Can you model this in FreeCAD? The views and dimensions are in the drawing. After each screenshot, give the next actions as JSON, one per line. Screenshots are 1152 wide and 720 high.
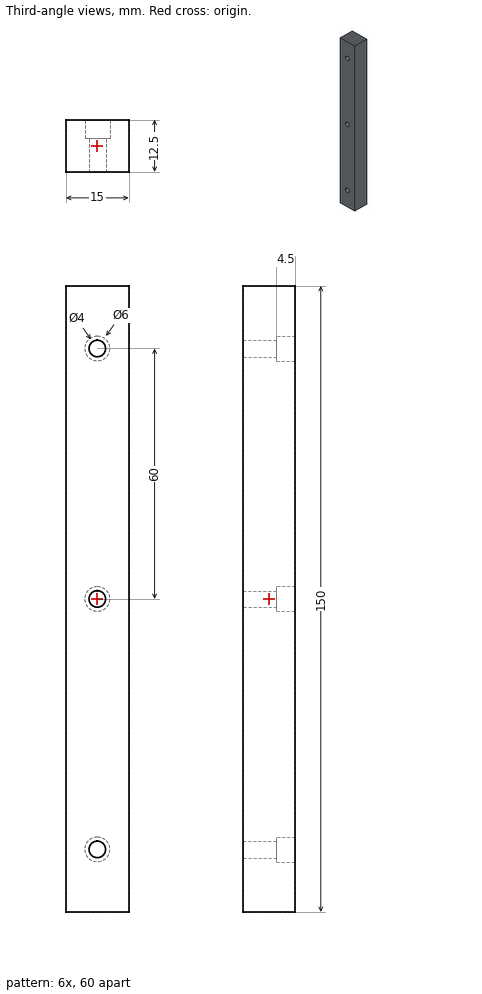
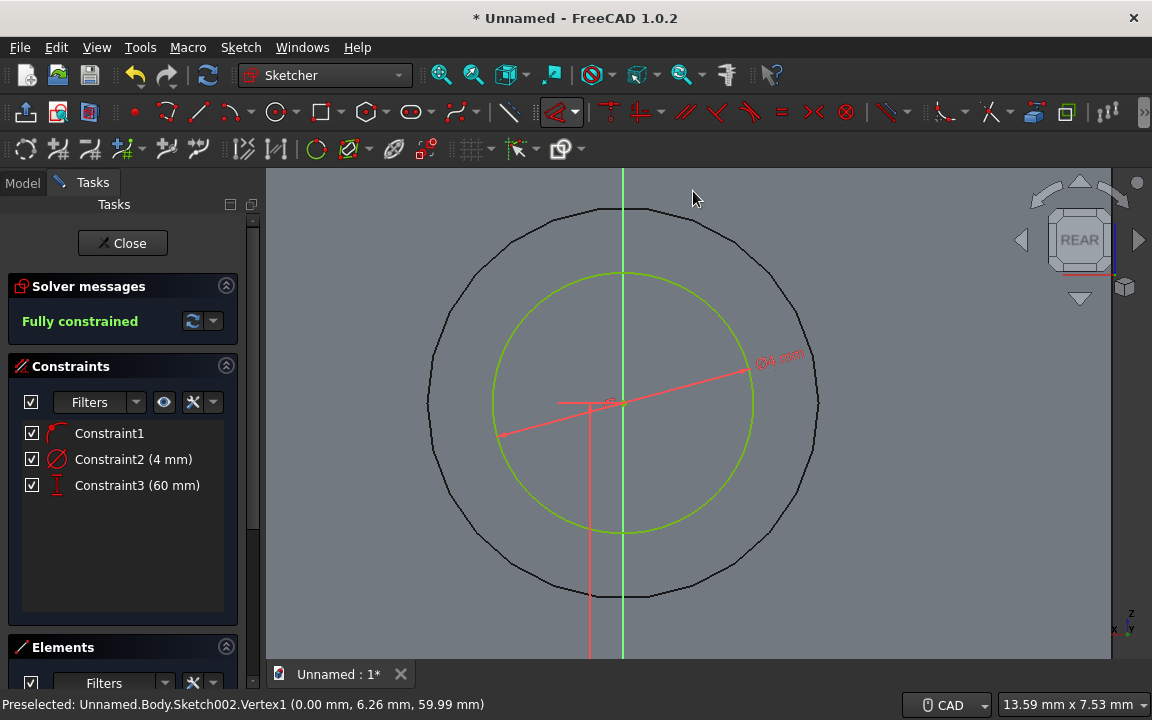
{"action": "left_click", "coordinate": [123, 243]}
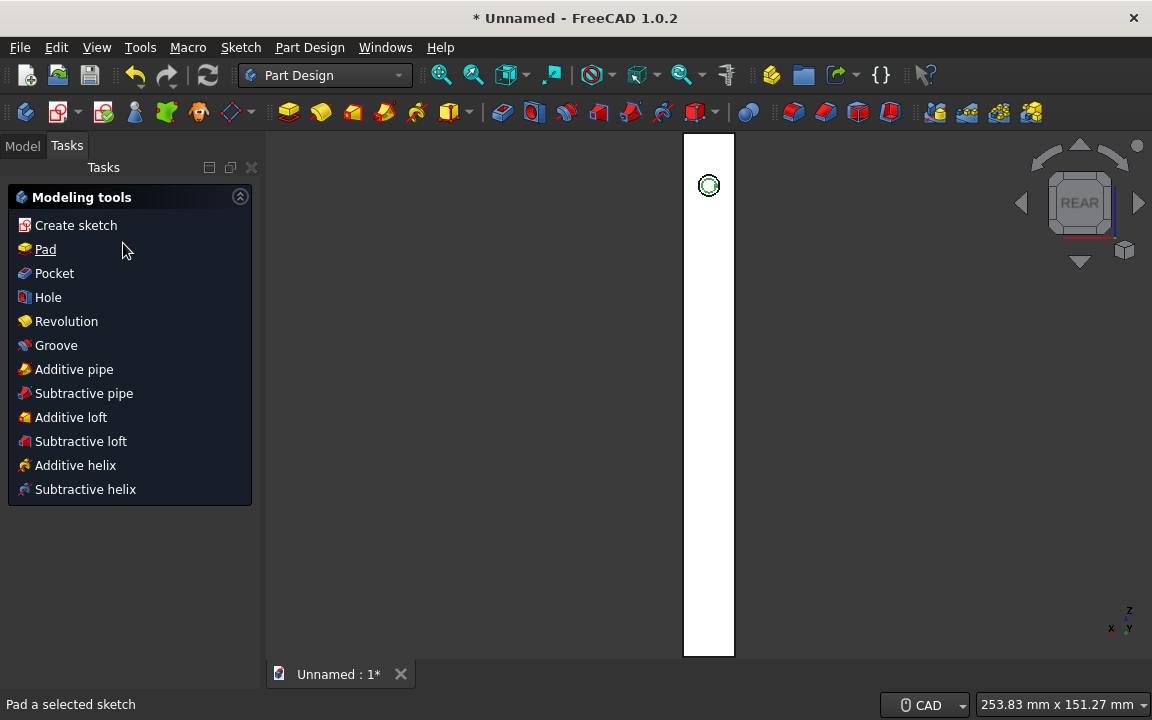
{"action": "left_click", "coordinate": [504, 112]}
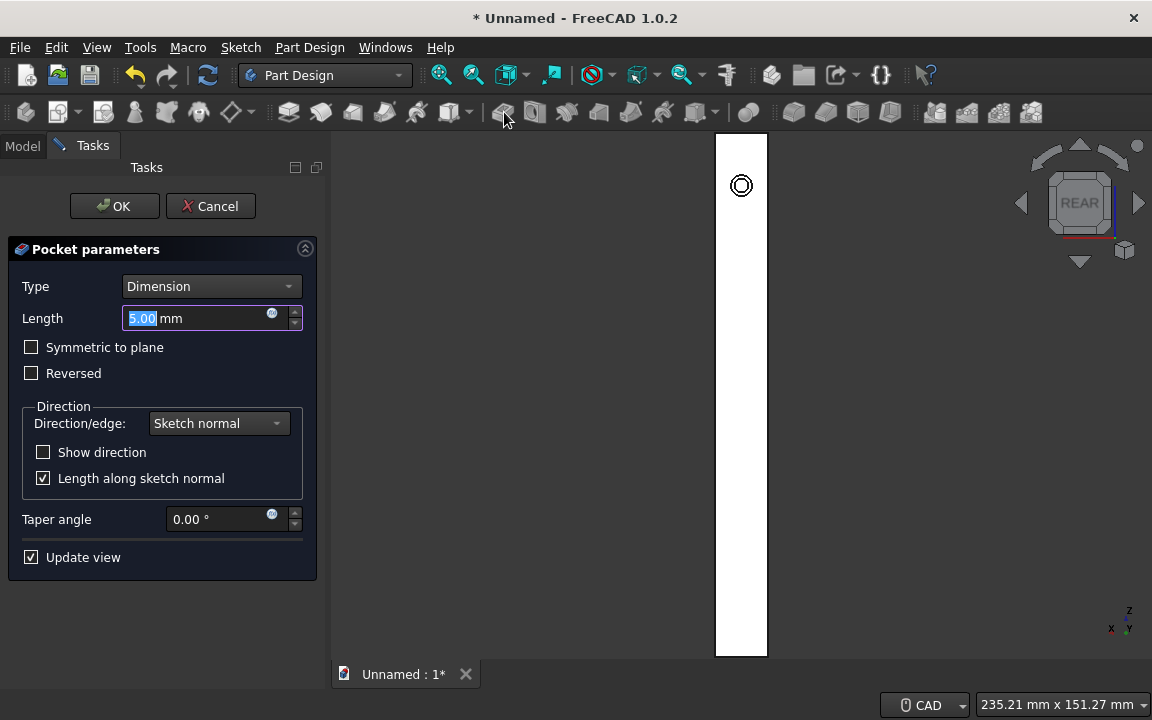
{"action": "left_click", "coordinate": [212, 286]}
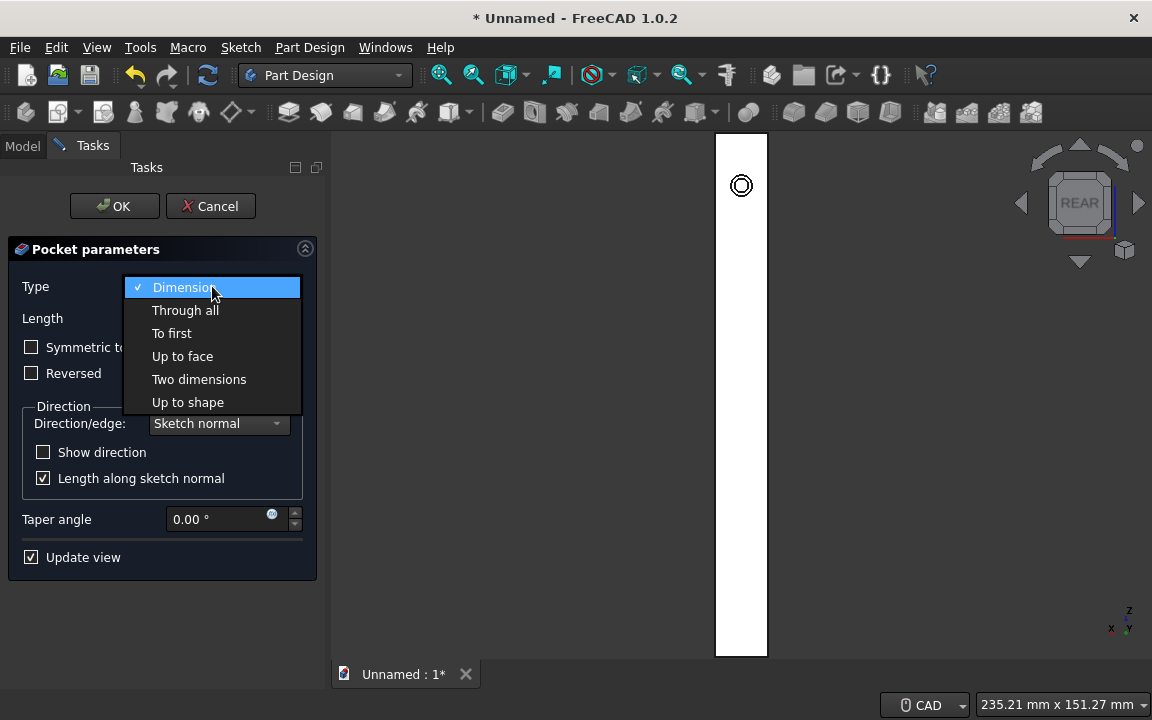
{"action": "left_click", "coordinate": [212, 310]}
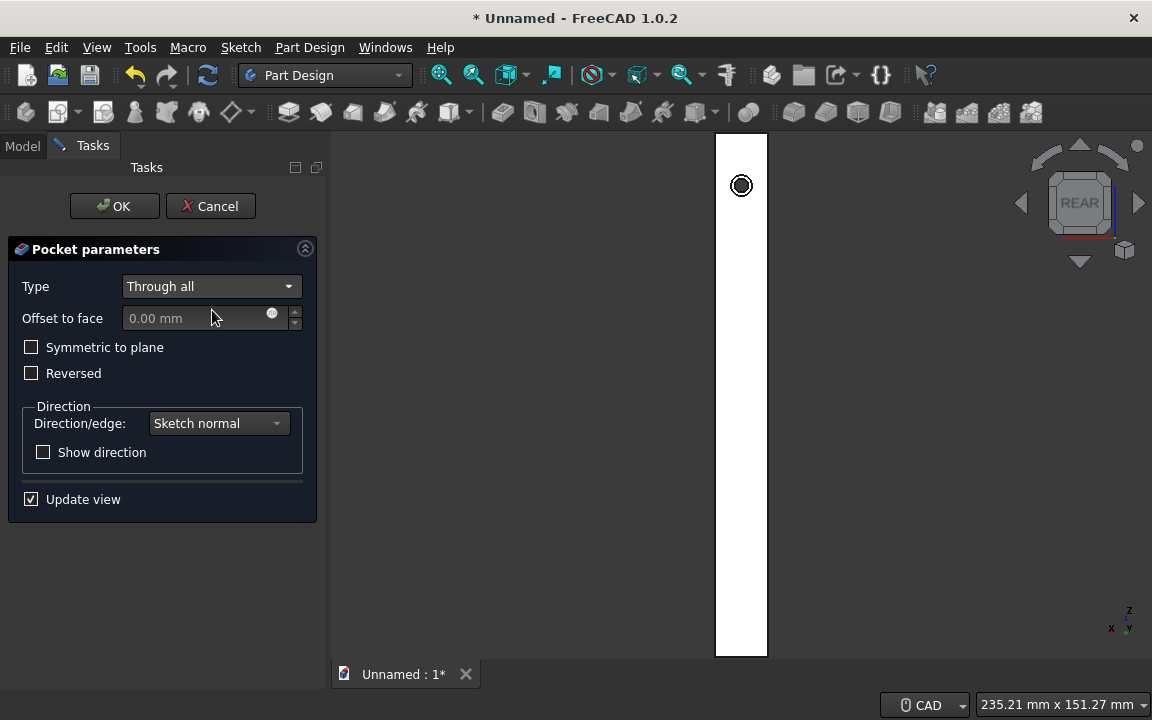
{"action": "left_click", "coordinate": [115, 206]}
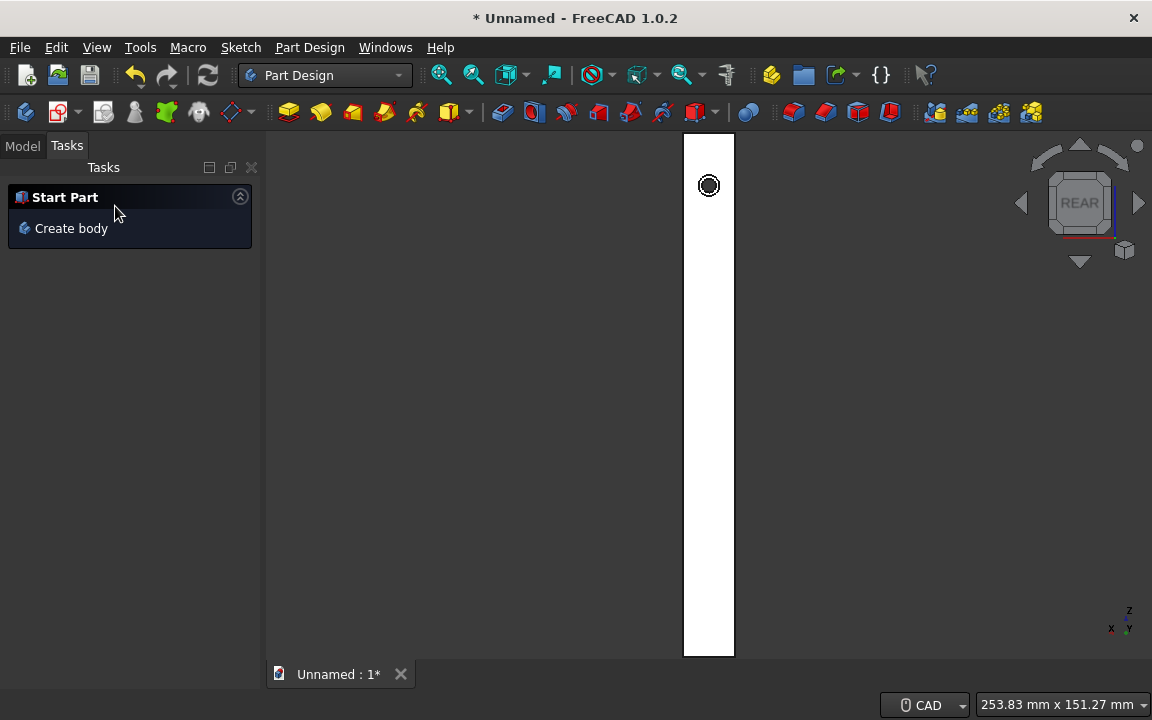
{"action": "left_click", "coordinate": [23, 145]}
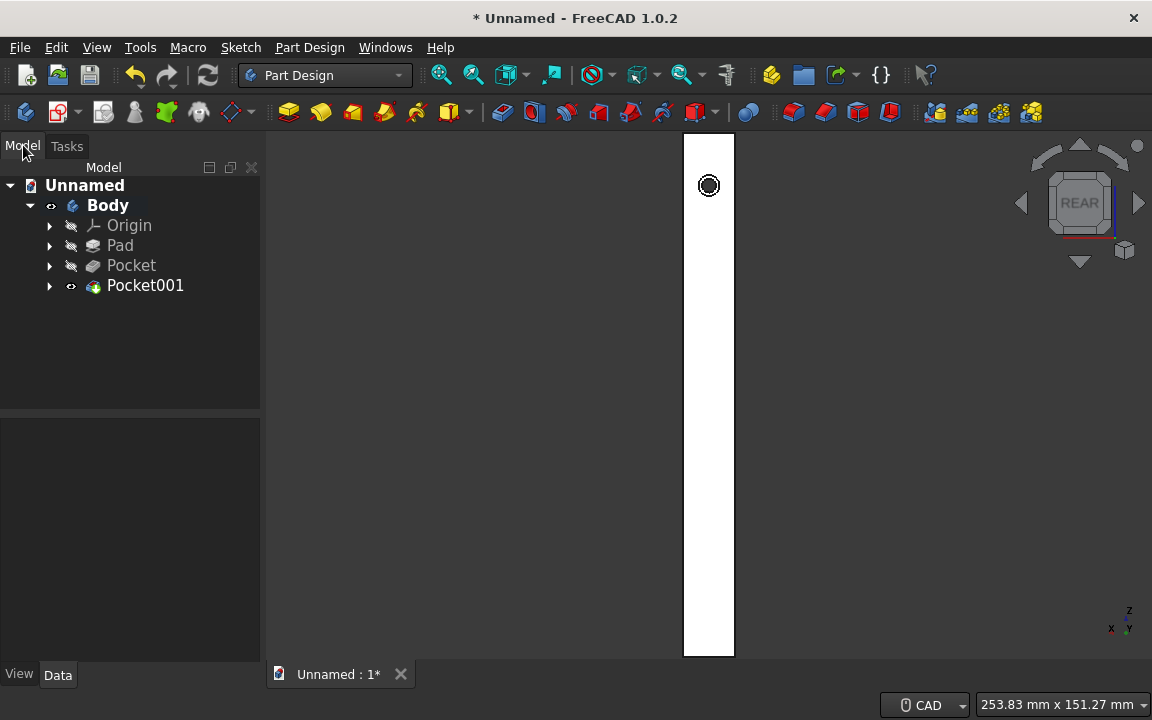
{"action": "left_click", "coordinate": [116, 266]}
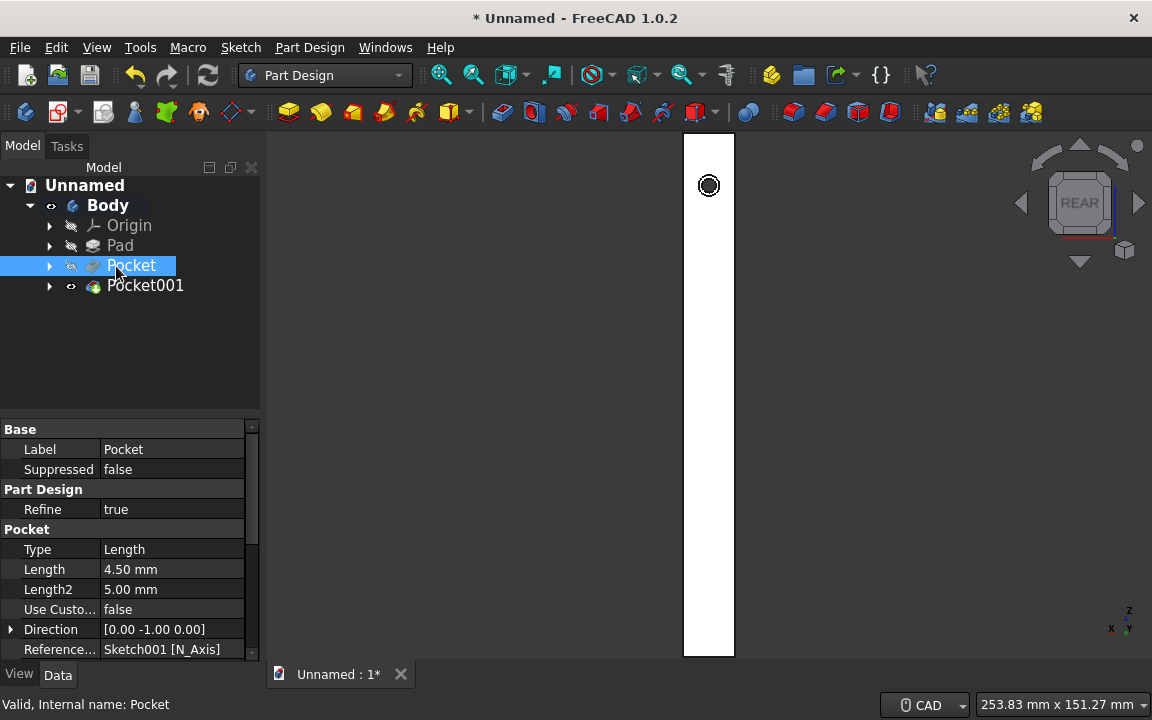
{"action": "left_click", "coordinate": [116, 286], "text": "ctrl"}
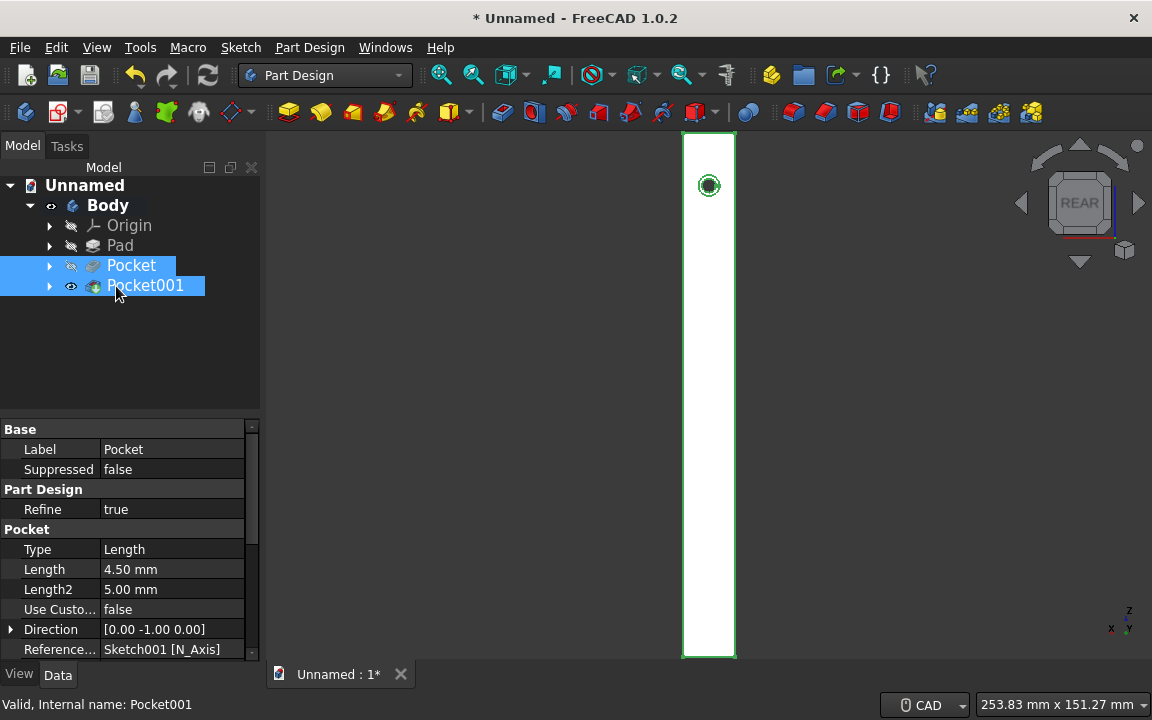
{"action": "left_click", "coordinate": [968, 112]}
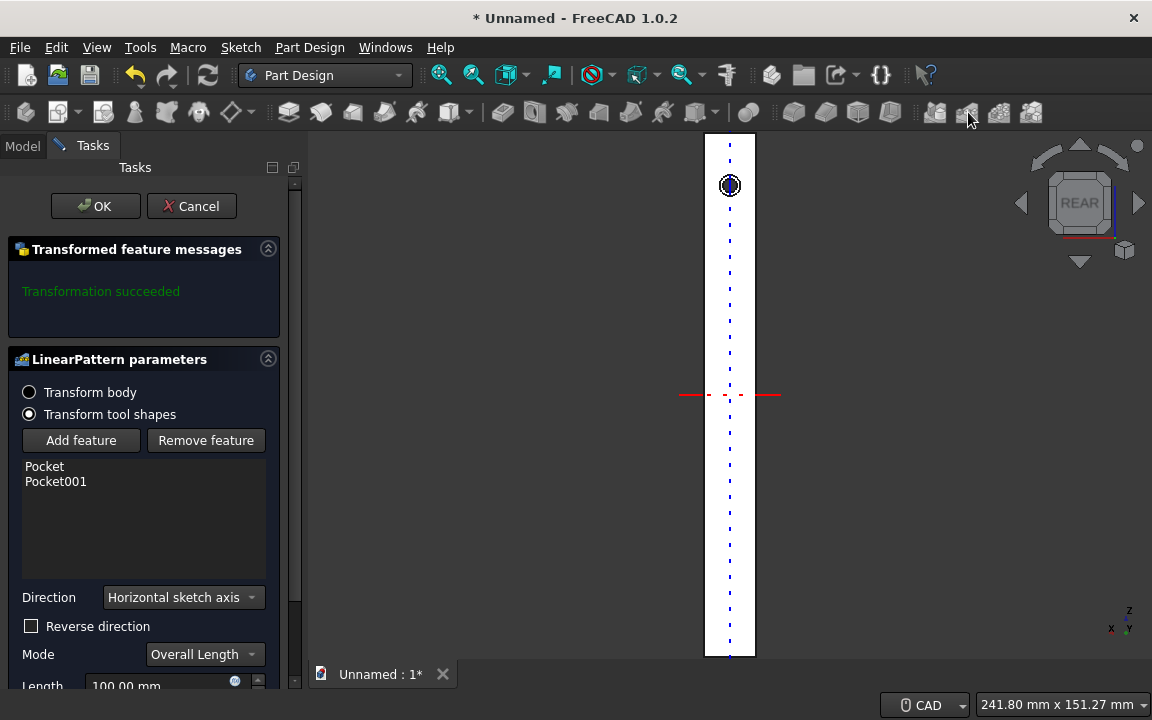
{"action": "left_click", "coordinate": [184, 598]}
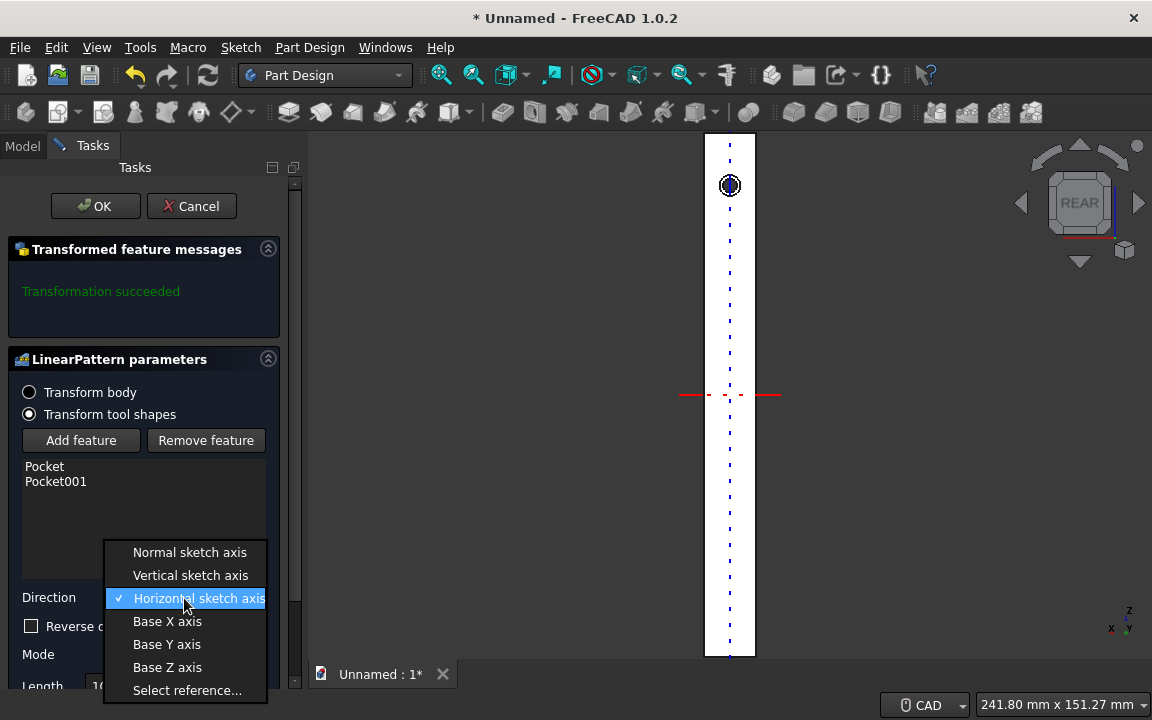
{"action": "left_click", "coordinate": [184, 668]}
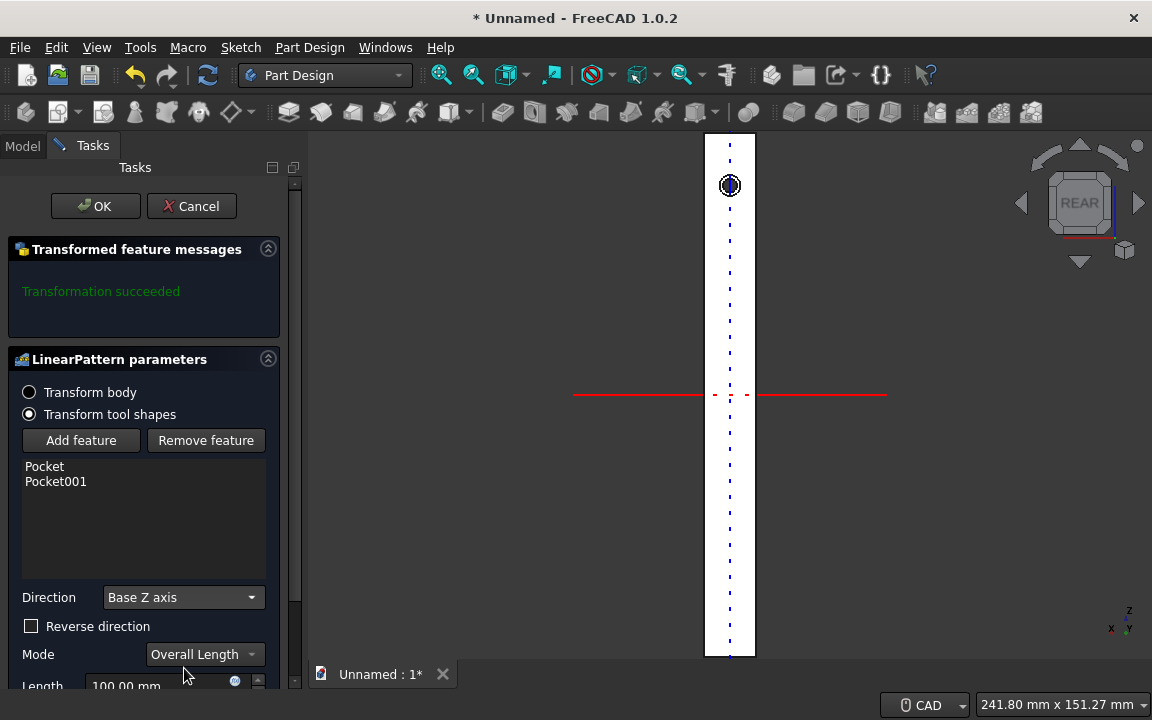
{"action": "left_click", "coordinate": [206, 654]}